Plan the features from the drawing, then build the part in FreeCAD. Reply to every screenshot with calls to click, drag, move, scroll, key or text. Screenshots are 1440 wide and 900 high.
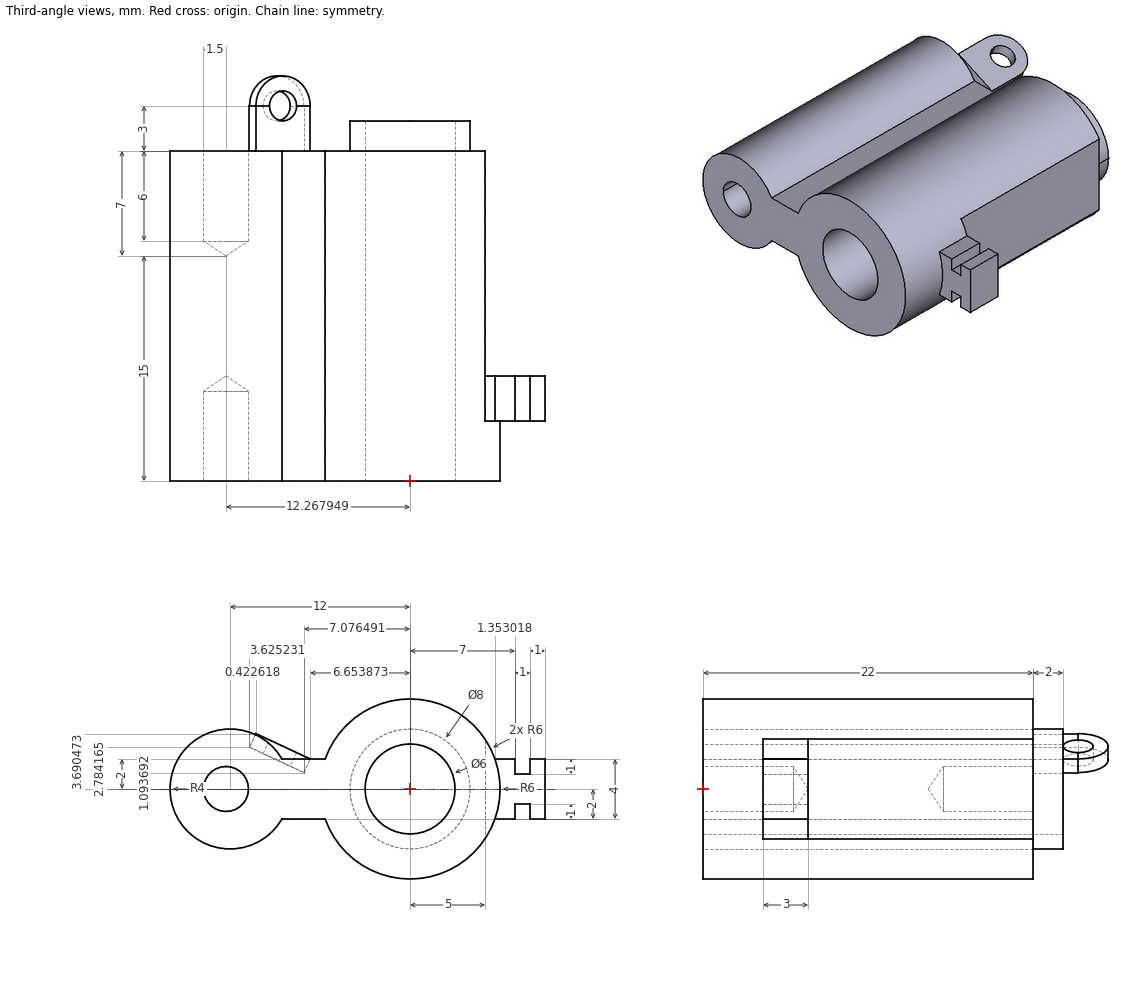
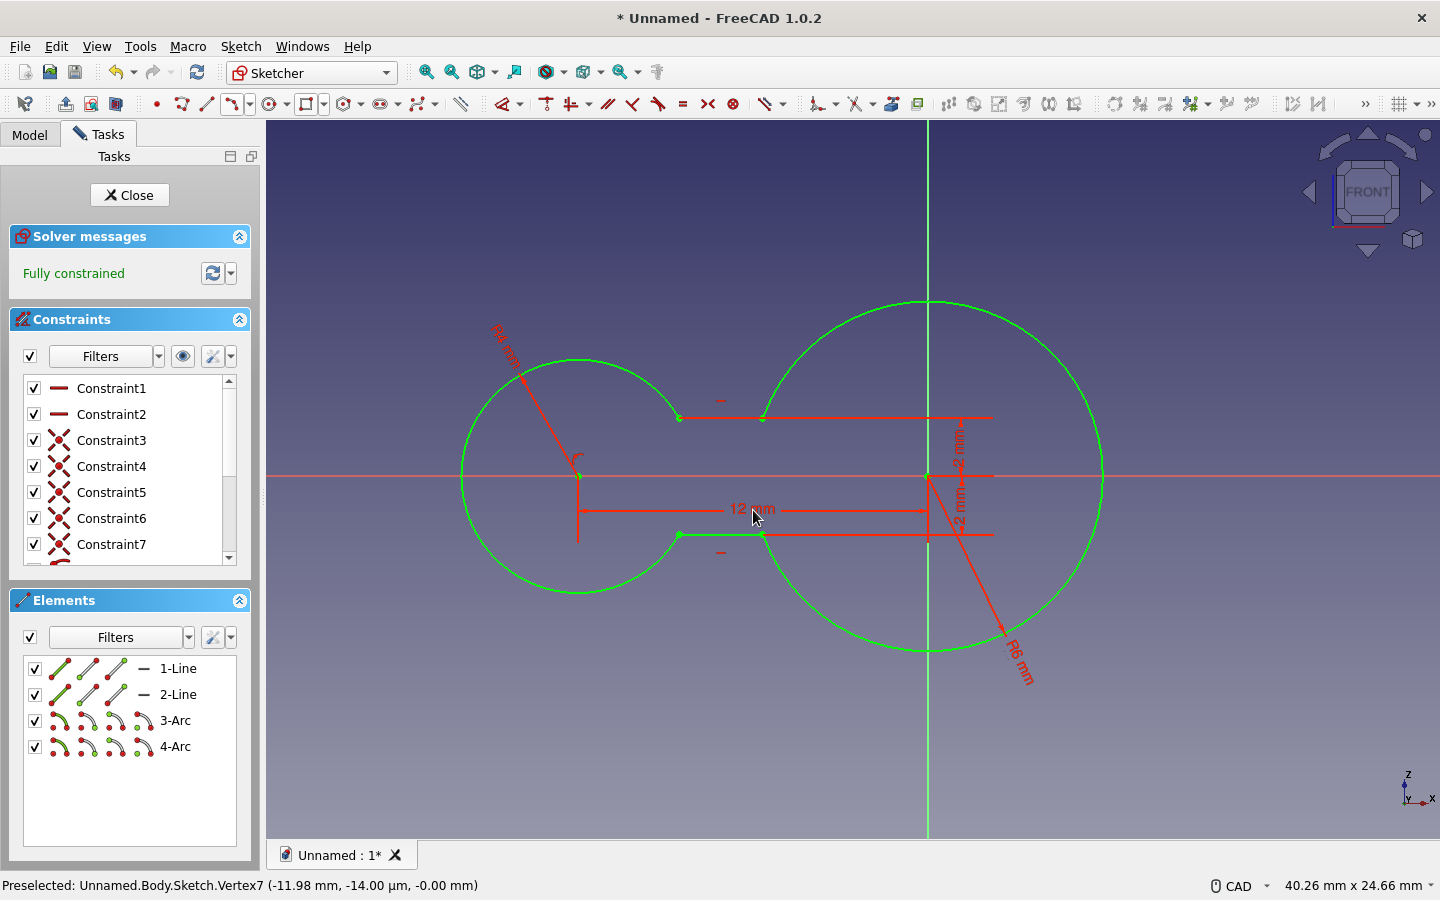
click(130, 195)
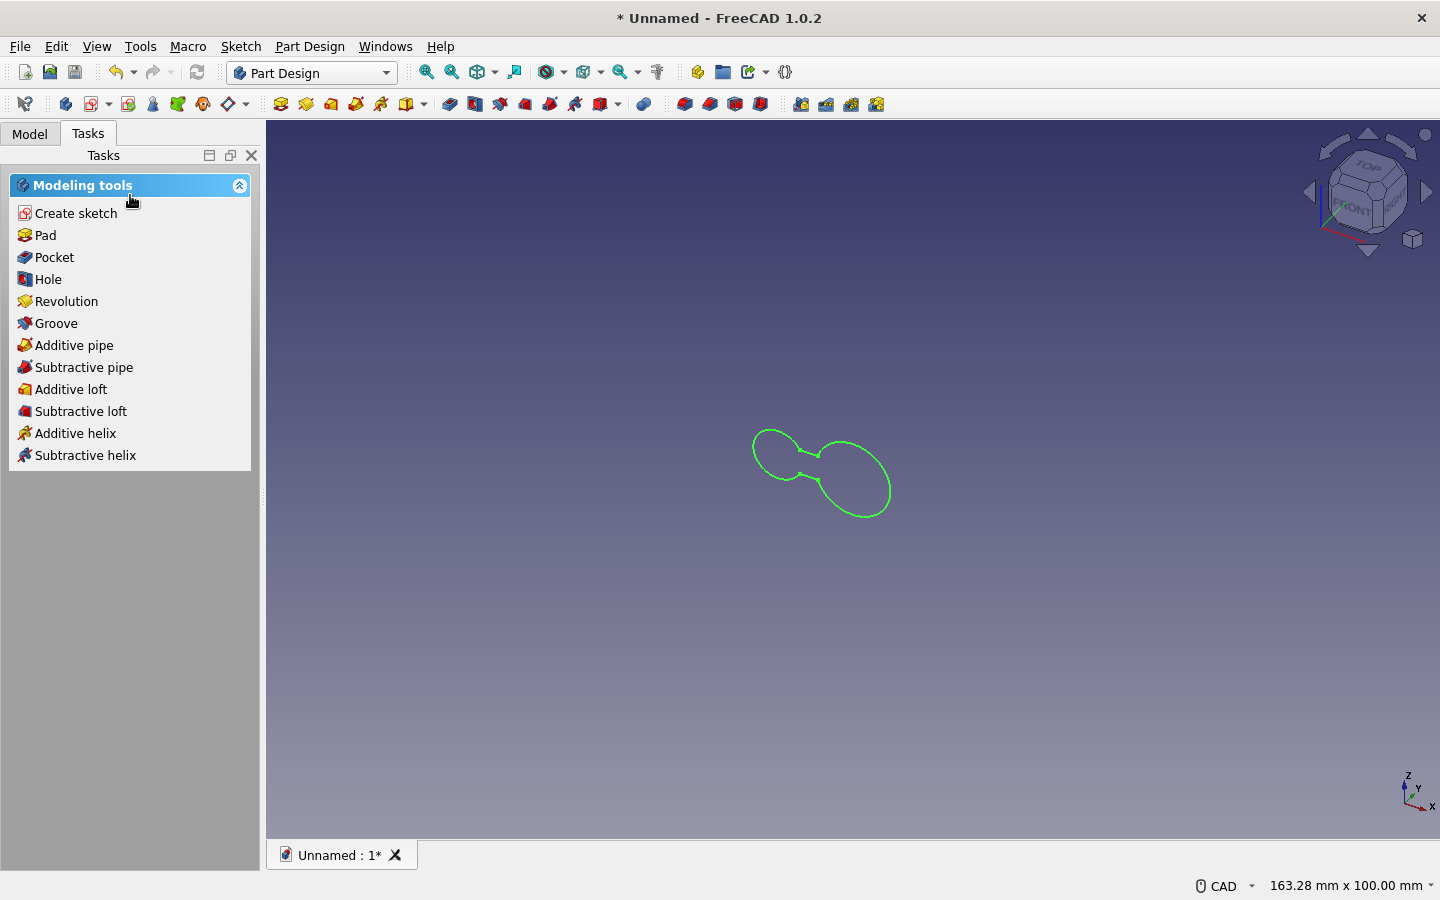
click(281, 104)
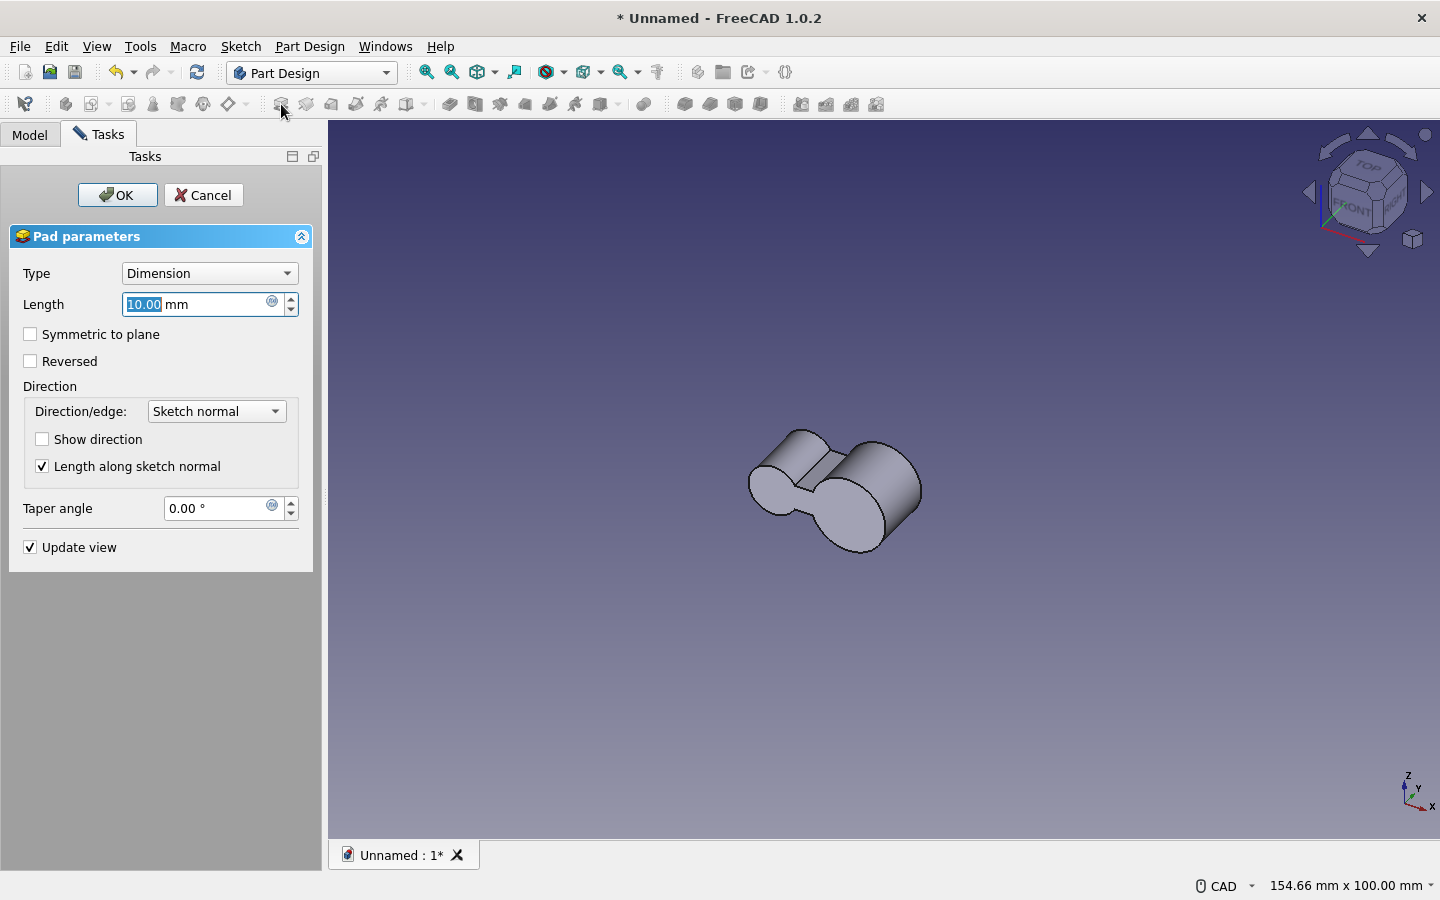
text(22)
key(Tab)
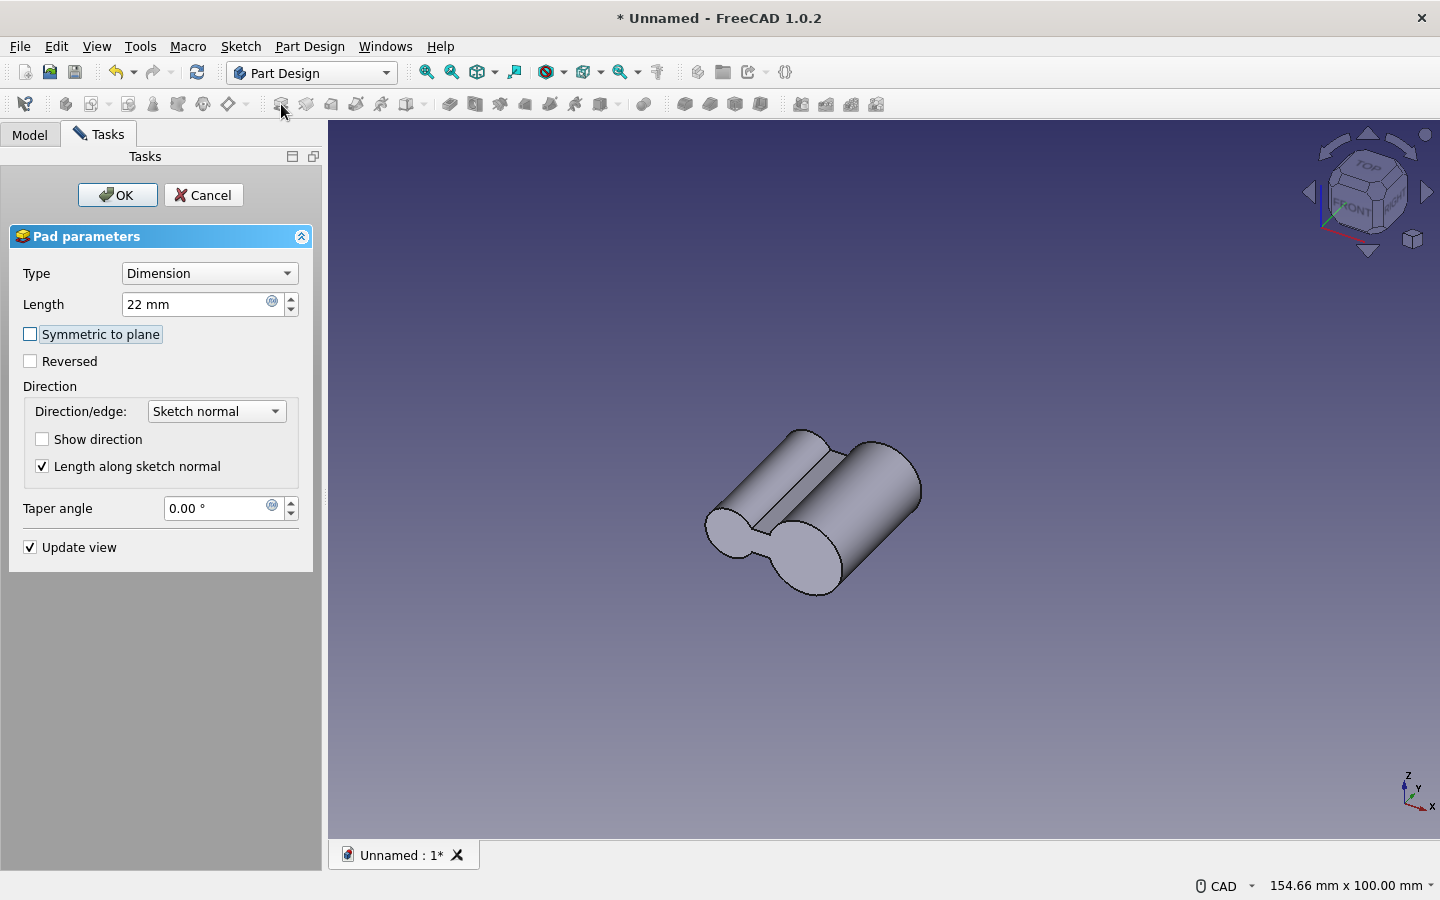
click(31, 361)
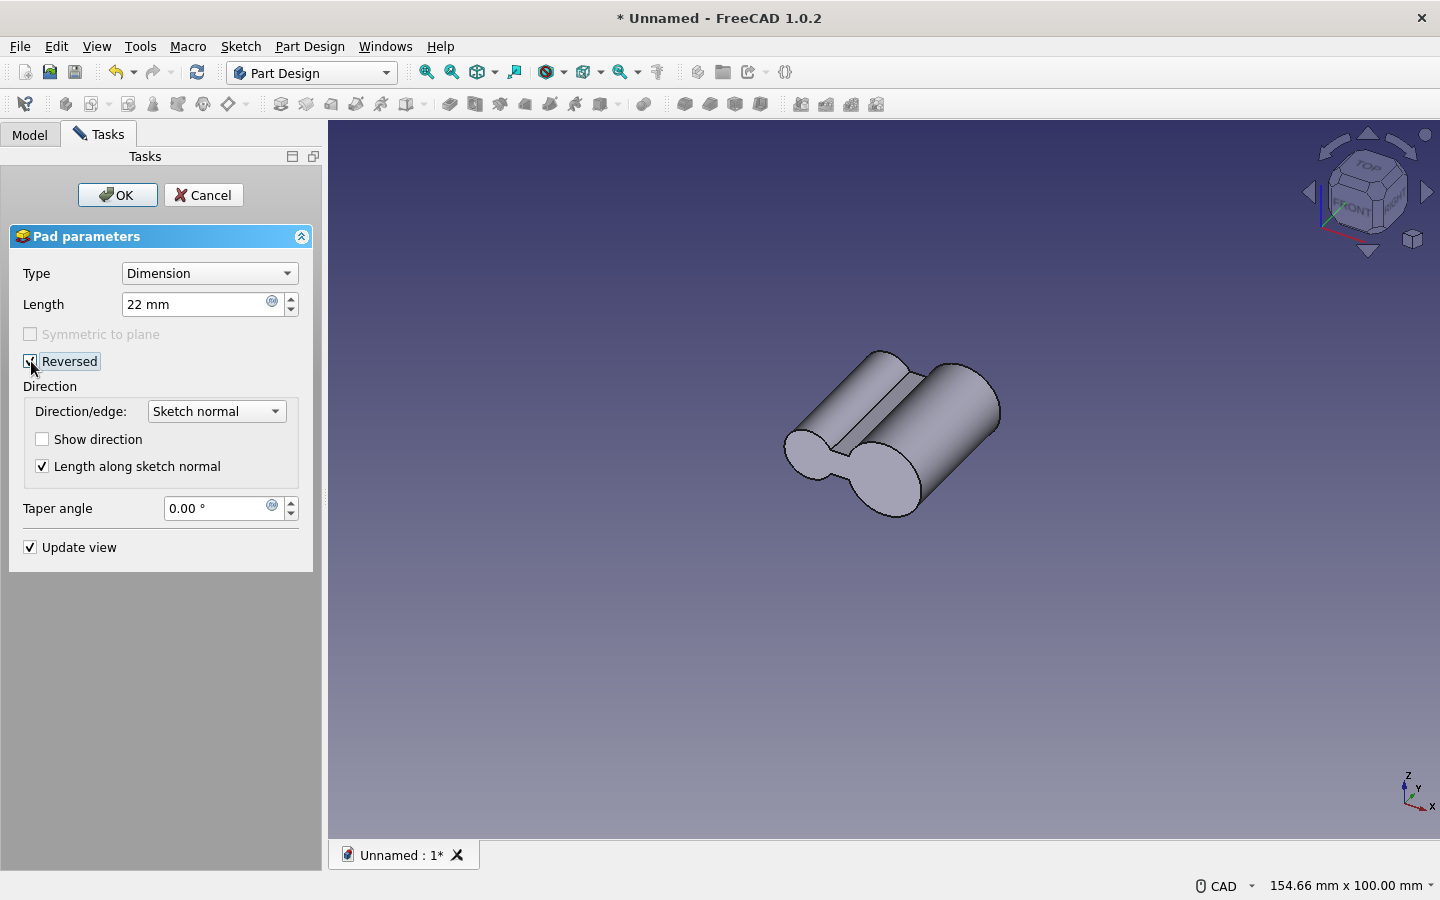
click(118, 195)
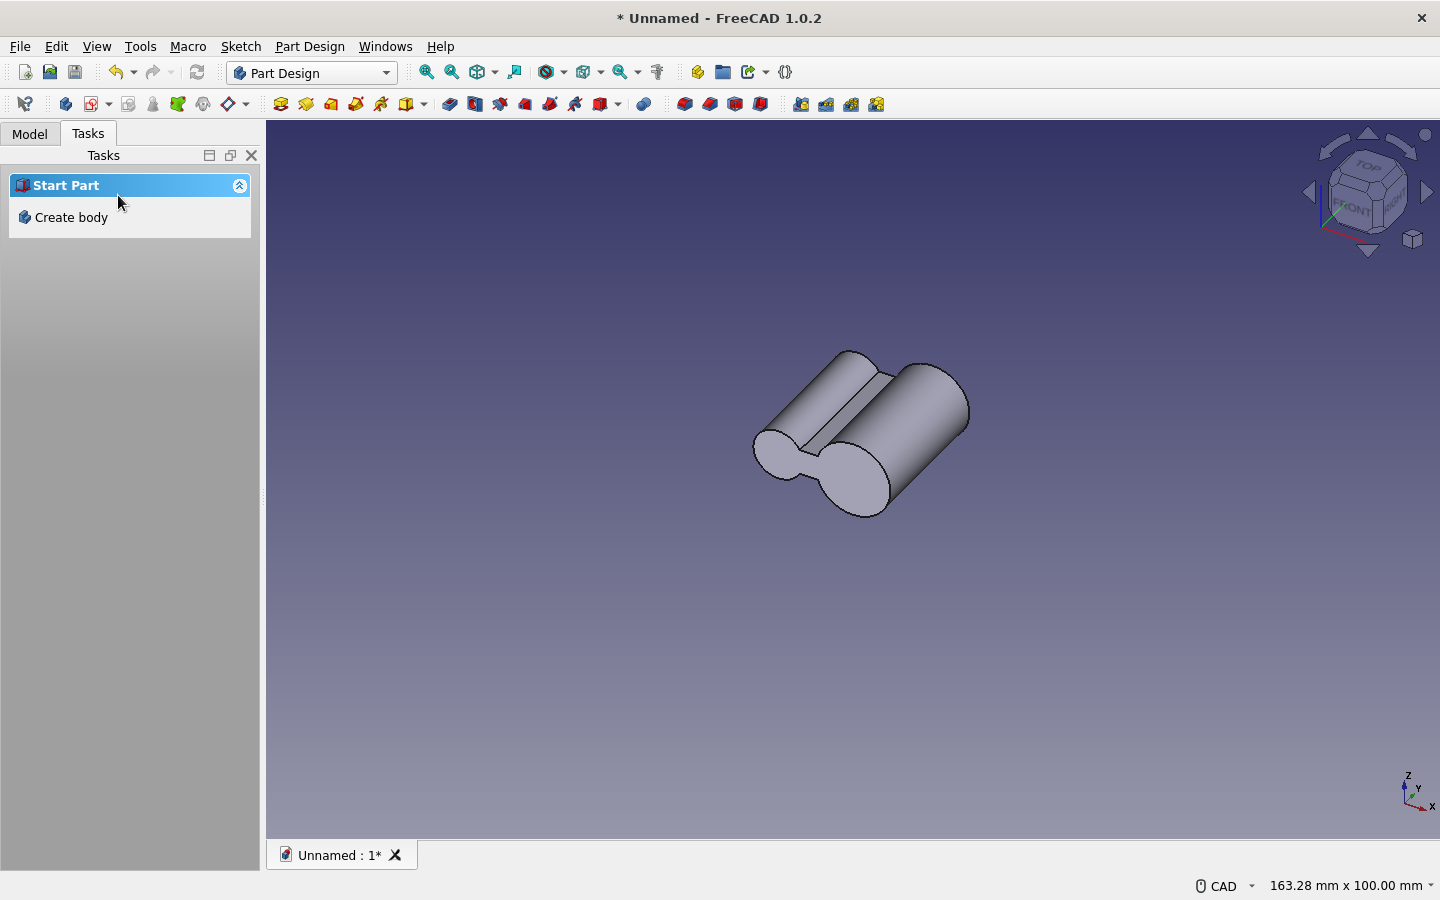
click(427, 72)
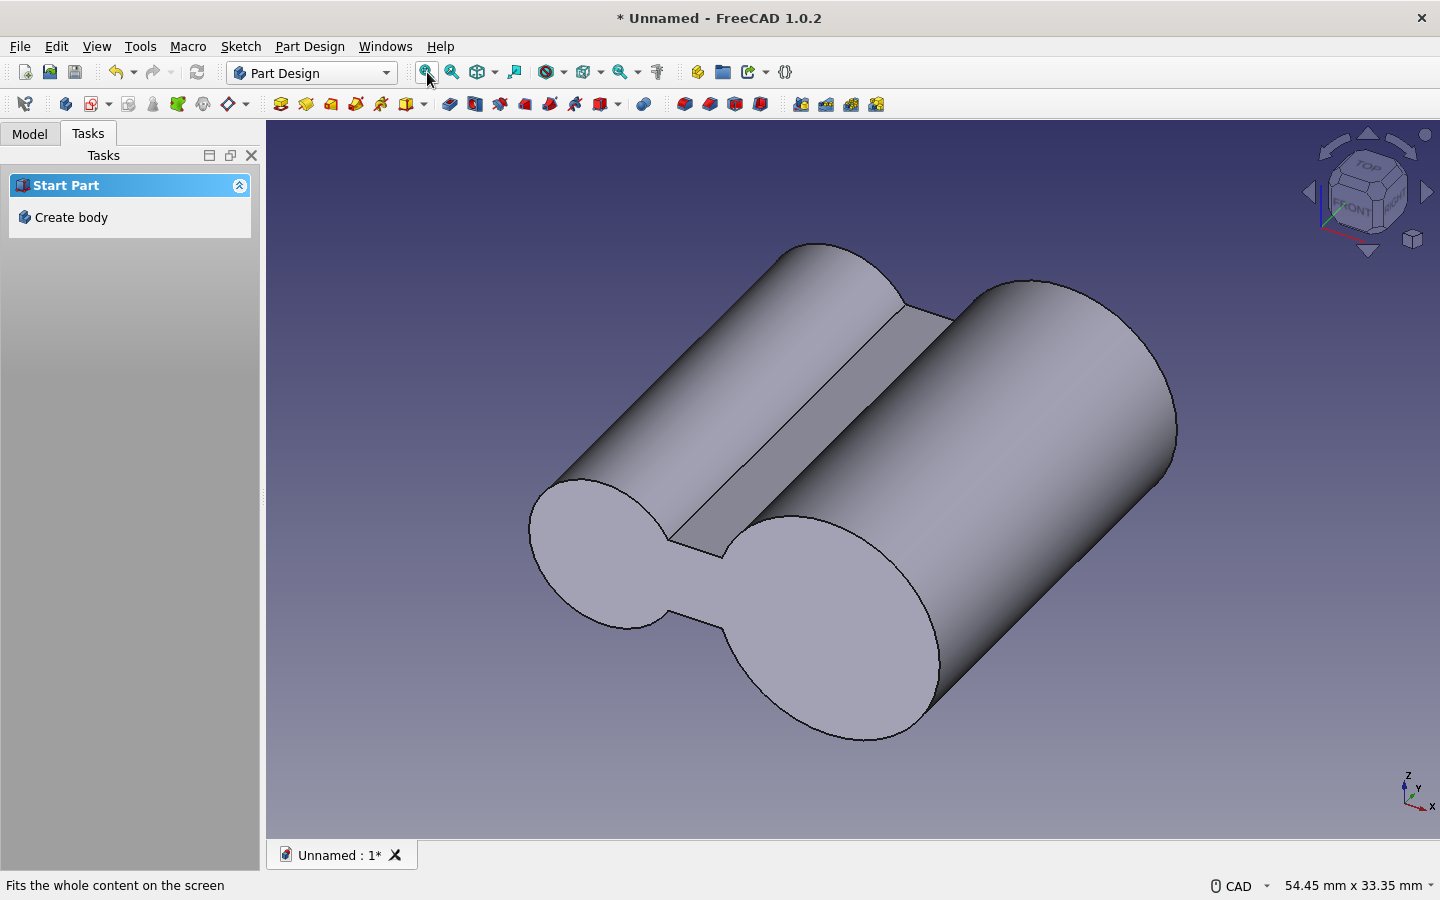
key(4)